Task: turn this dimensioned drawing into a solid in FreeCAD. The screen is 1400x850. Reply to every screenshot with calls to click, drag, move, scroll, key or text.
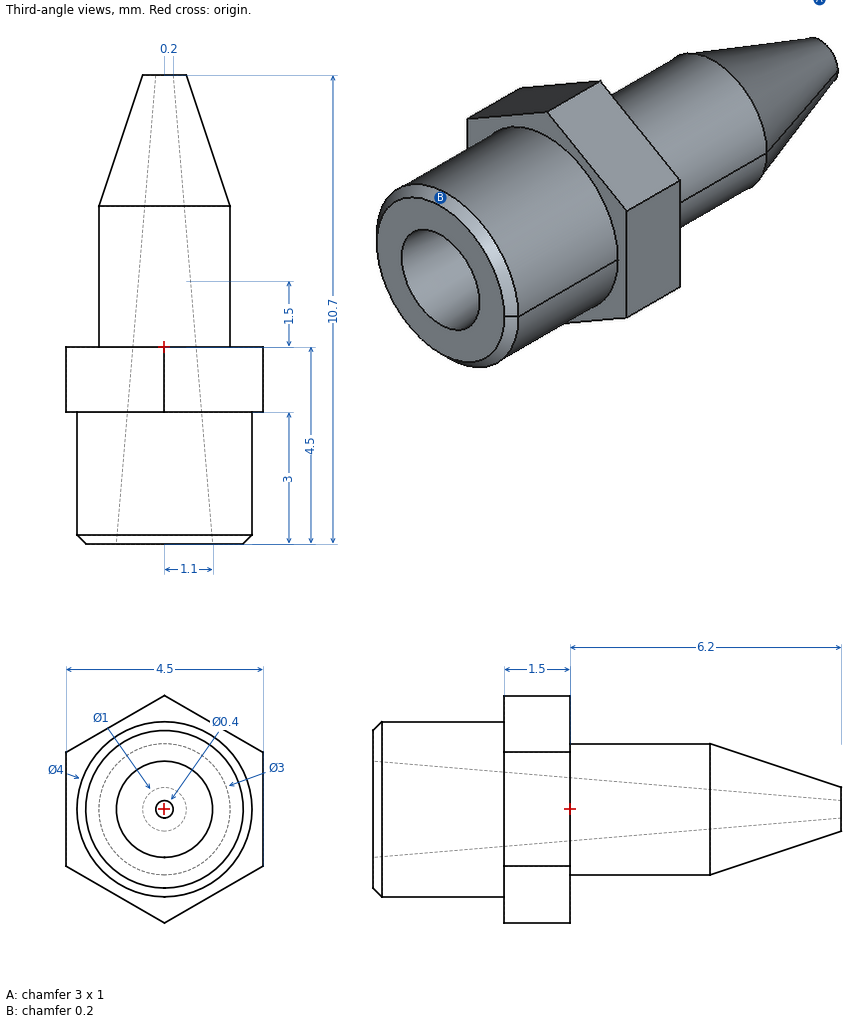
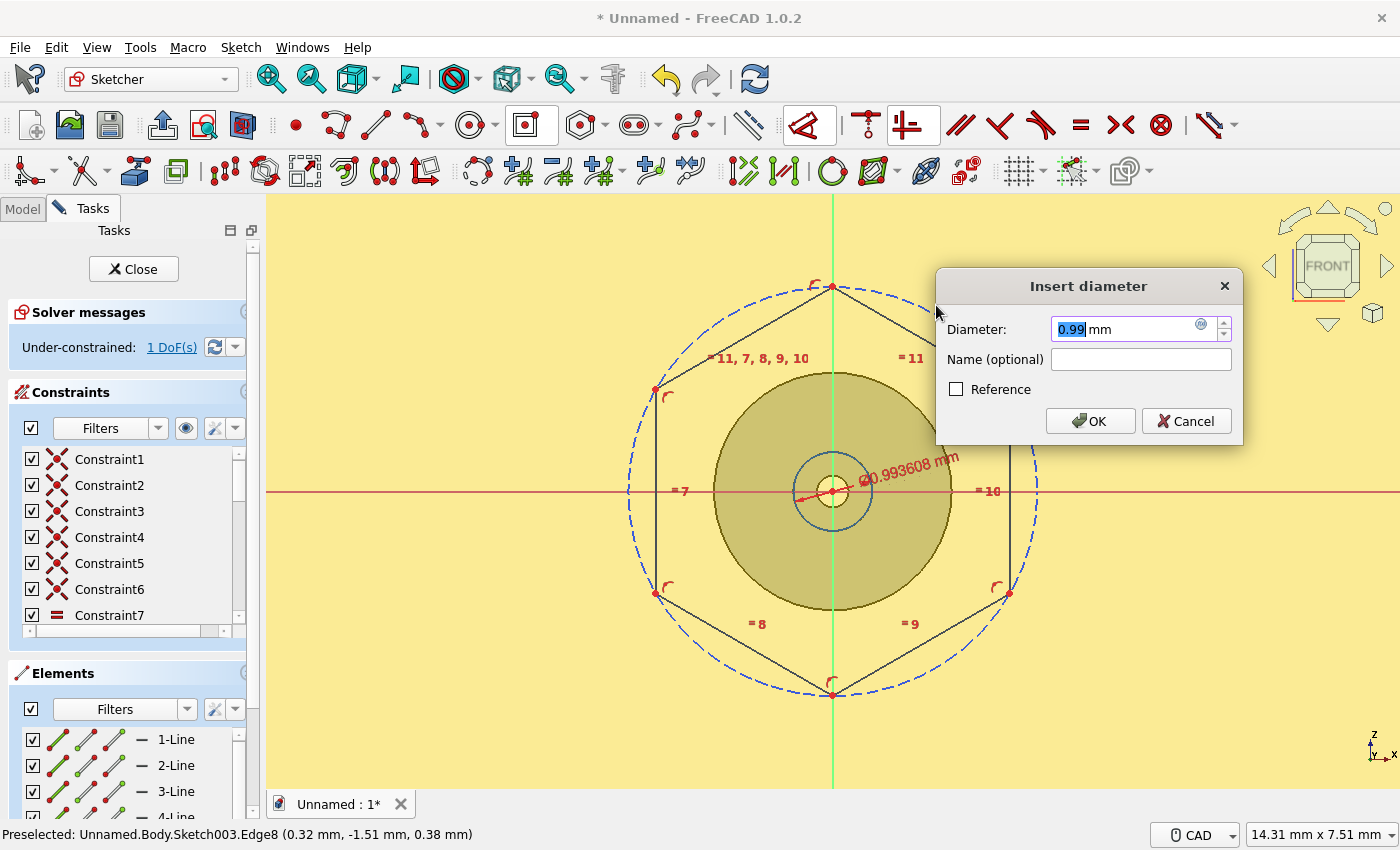
text(1)
key(Return)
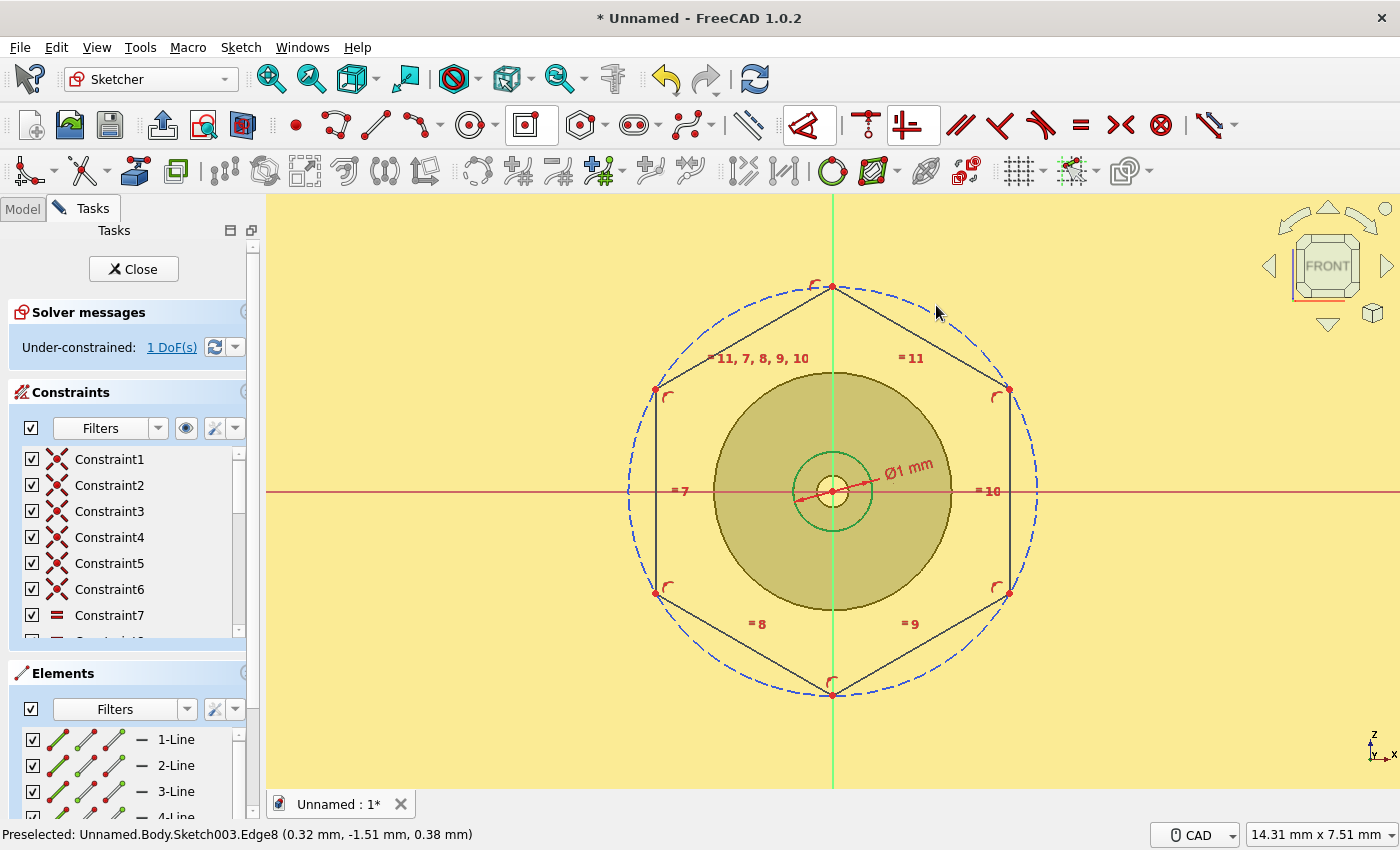
click(656, 389)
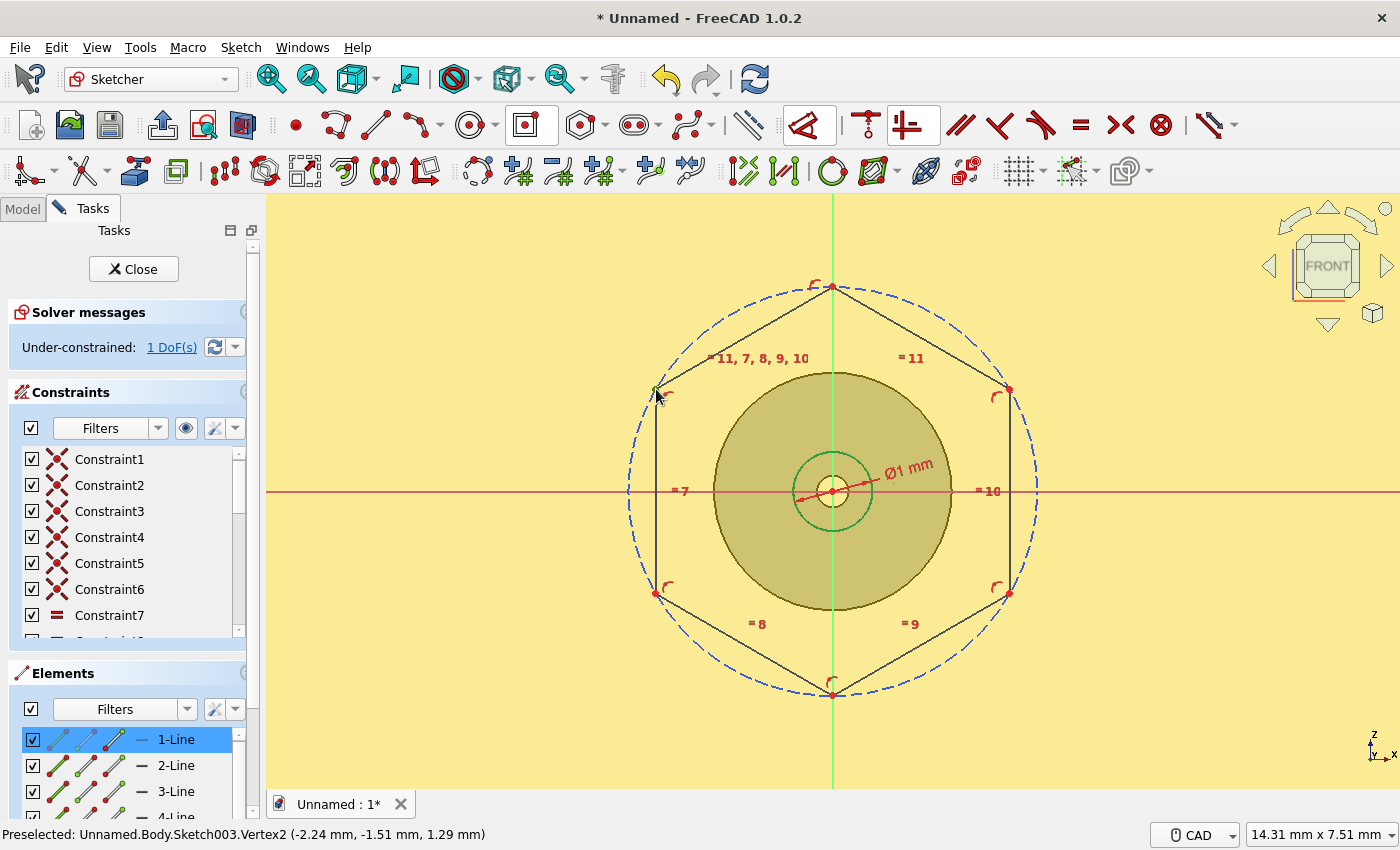
click(1010, 594)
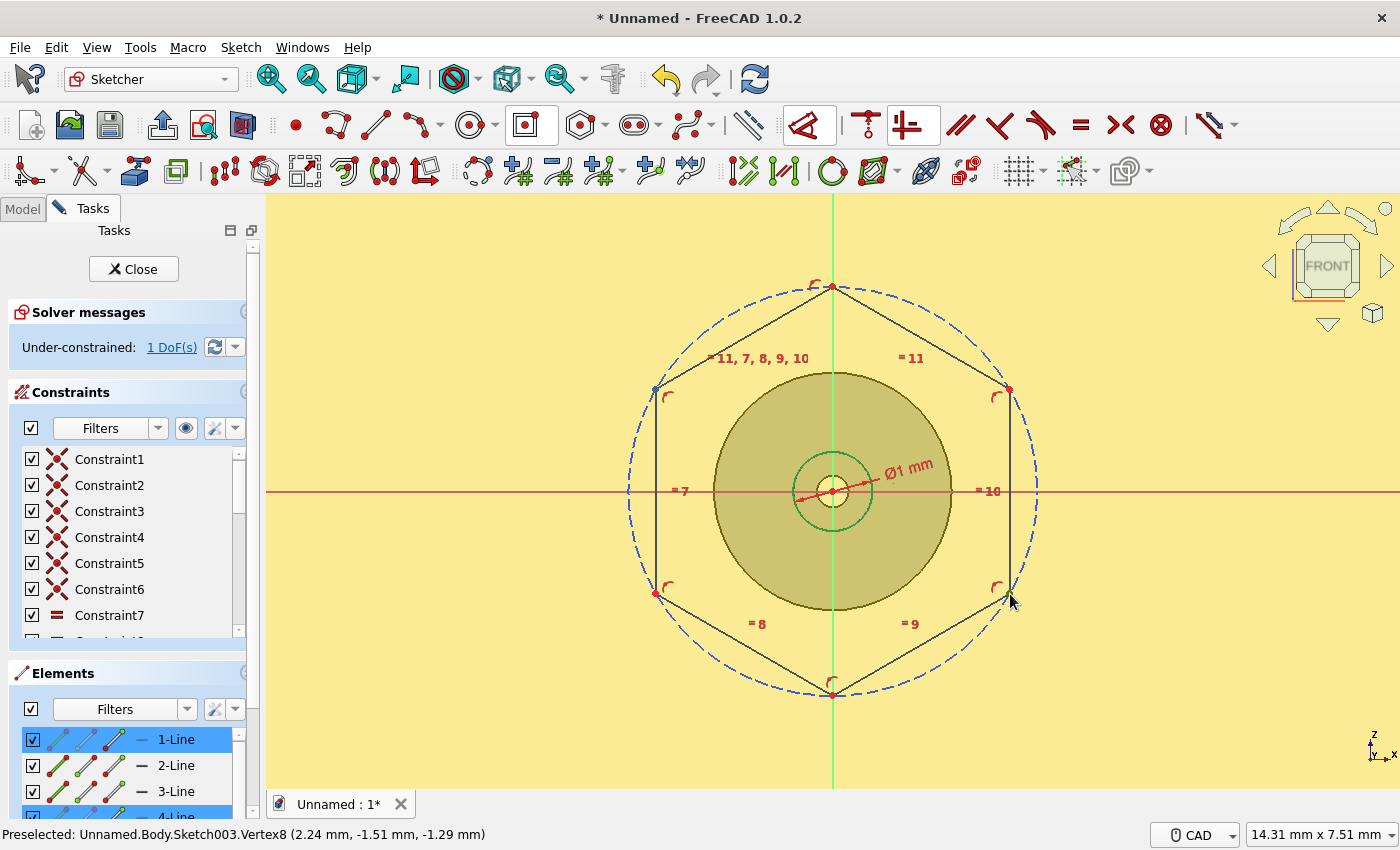
key(l)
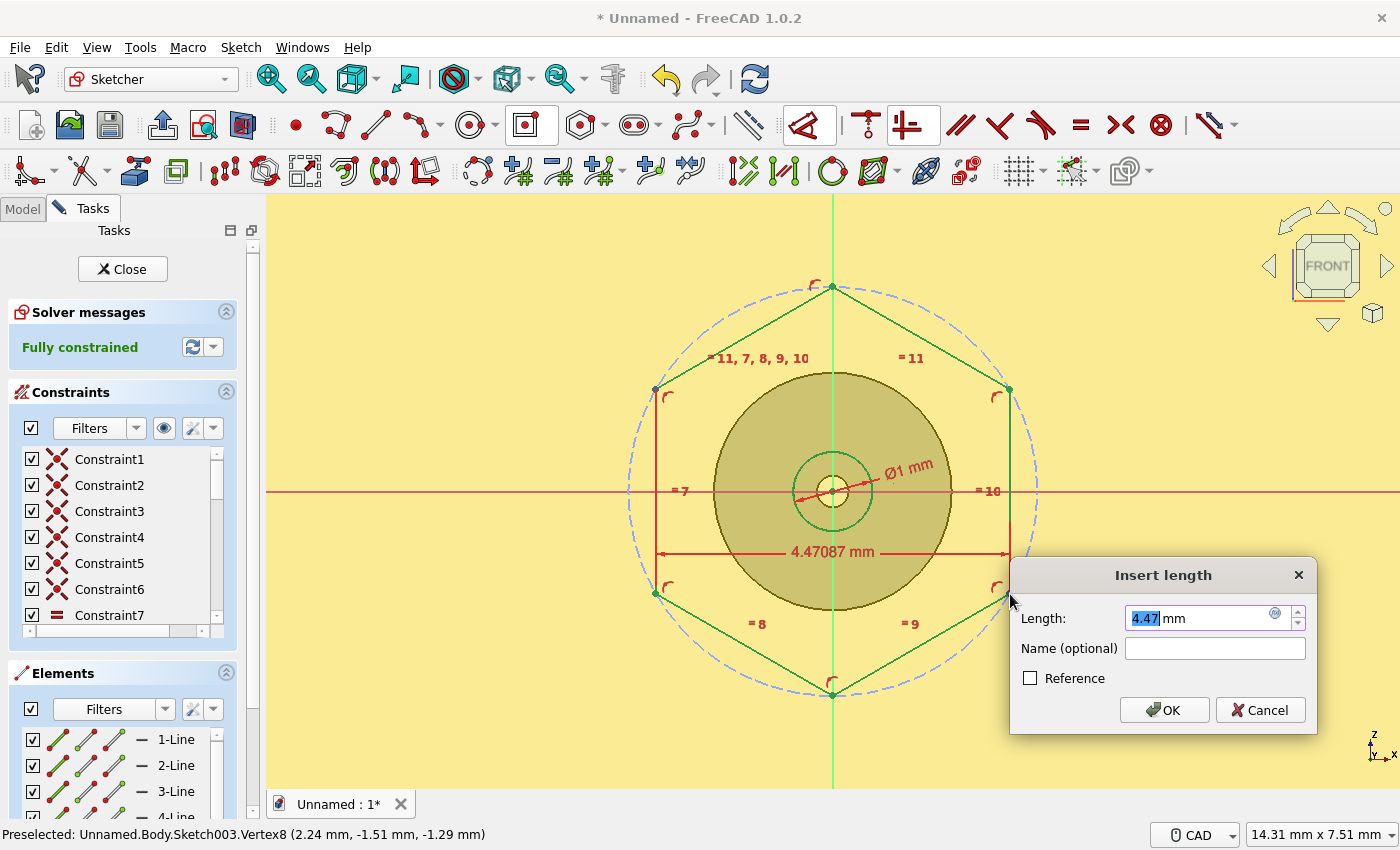
text(4.5)
key(Return)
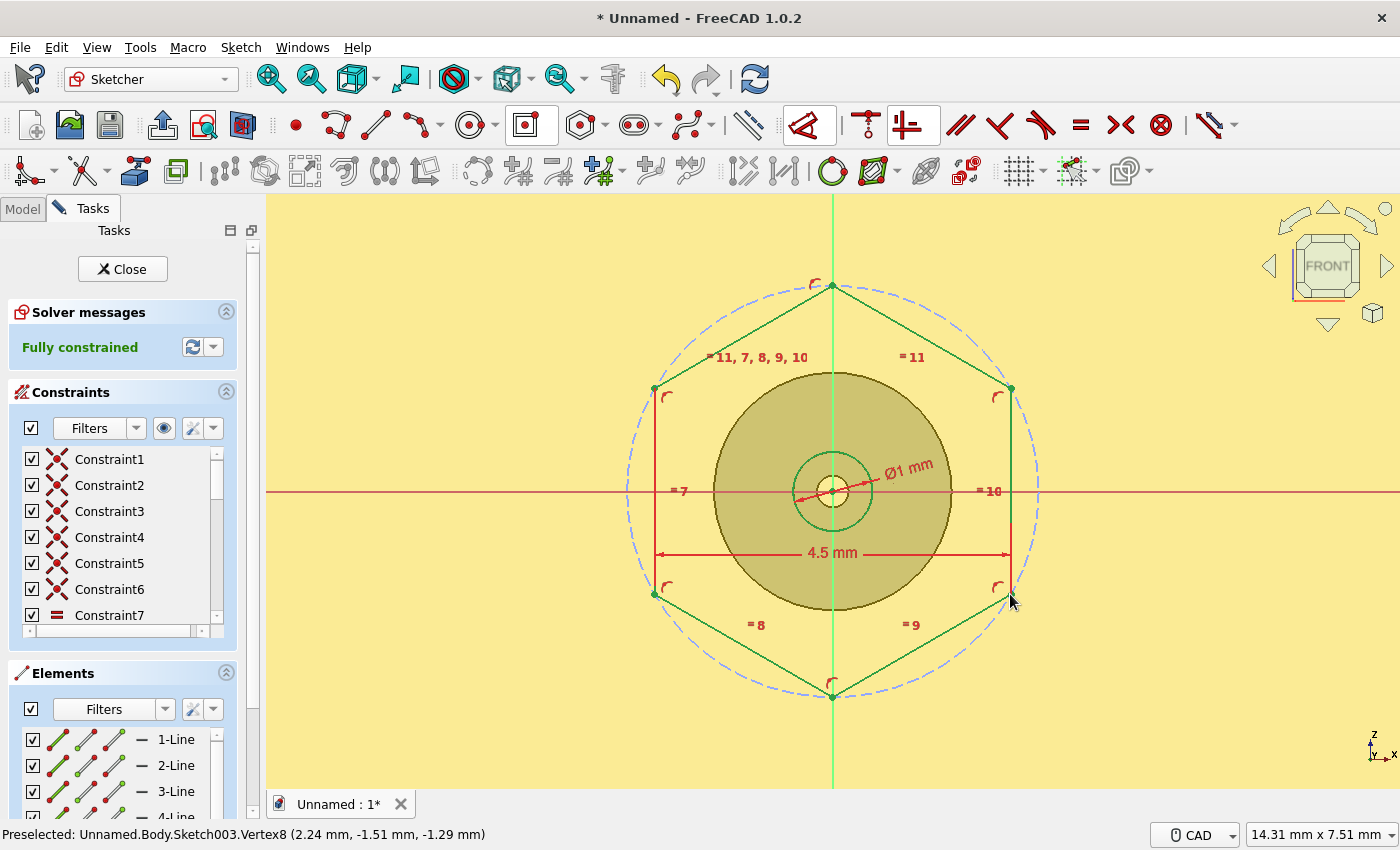
click(123, 269)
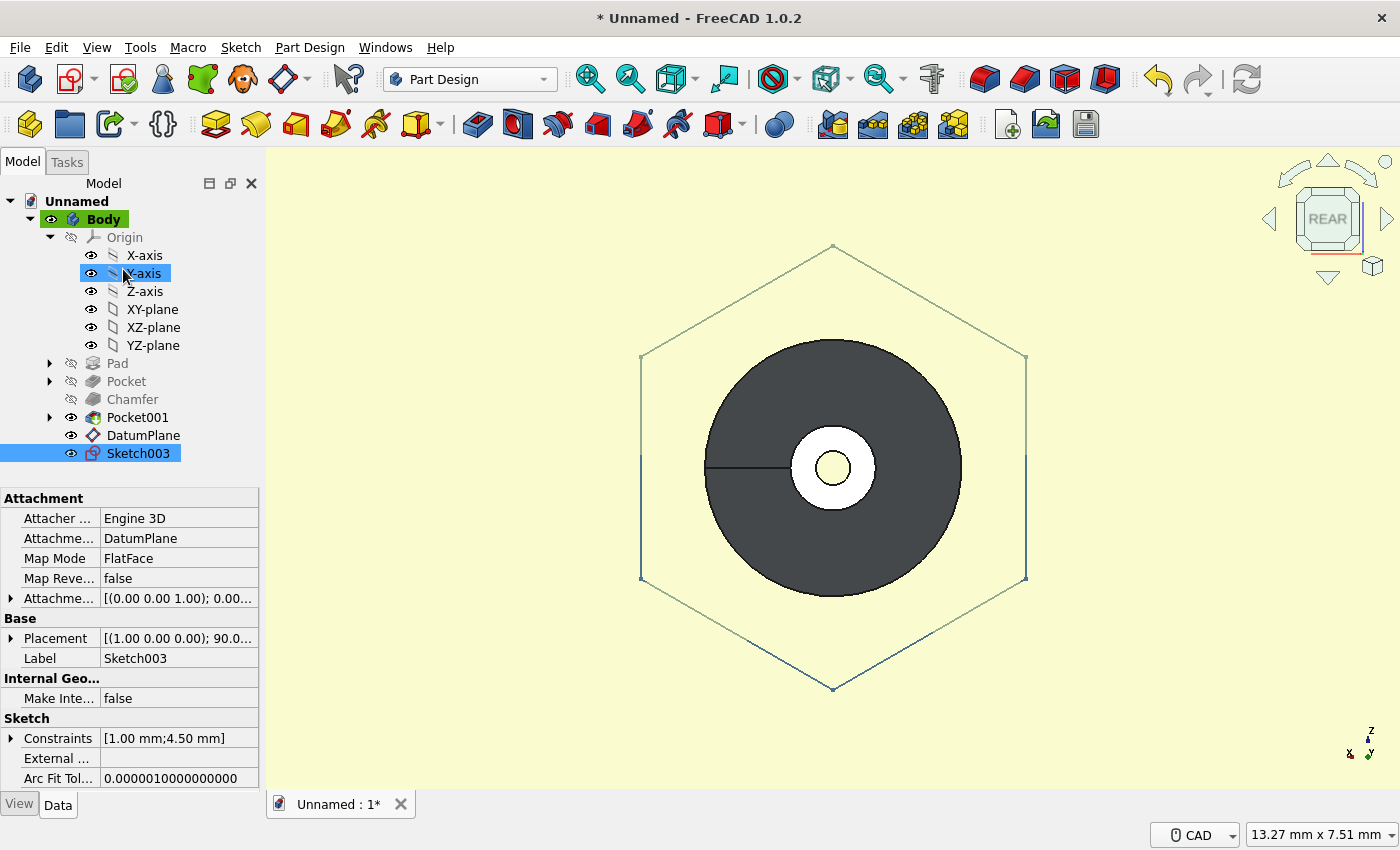
click(216, 124)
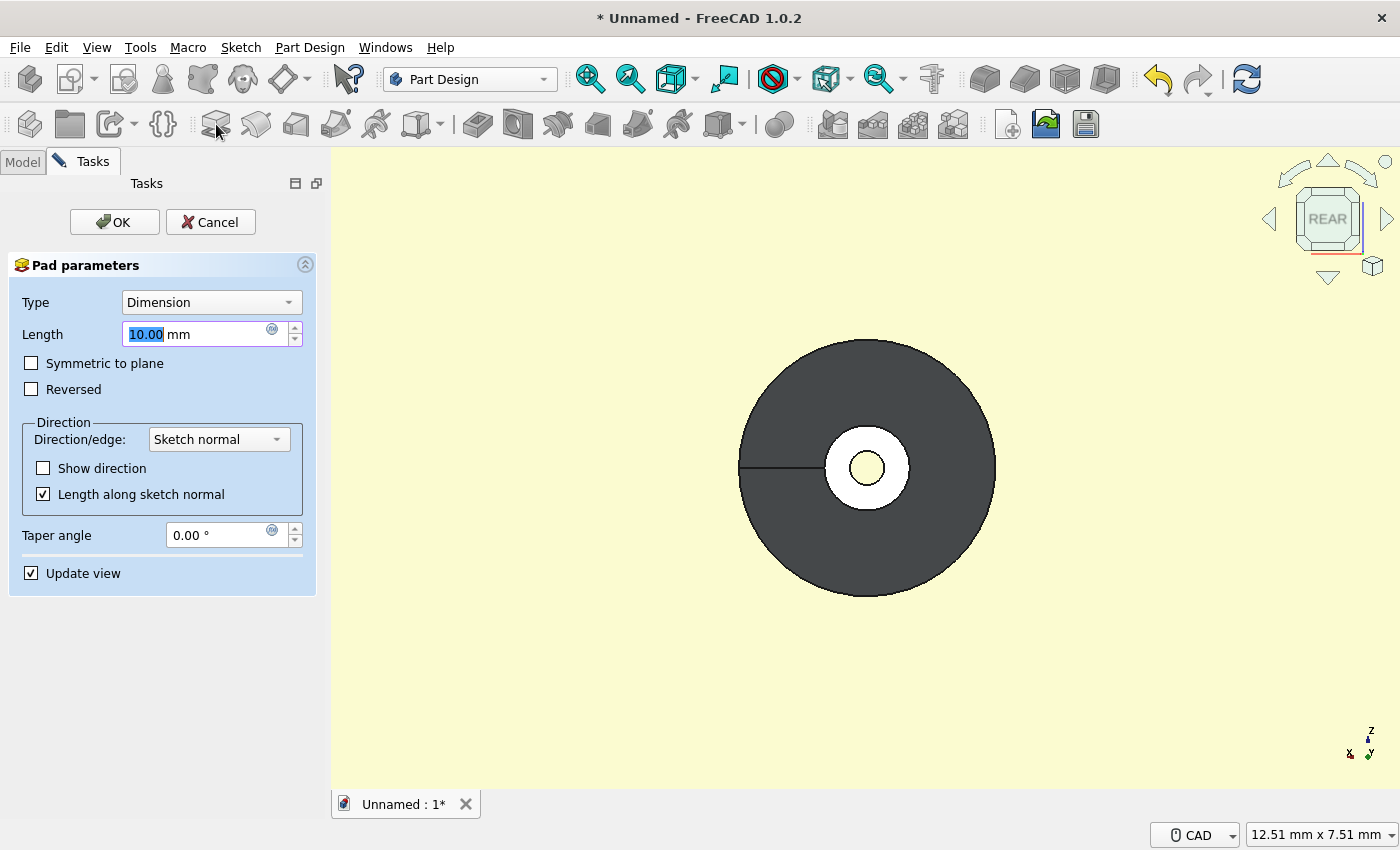
text(1.5)
key(Tab)